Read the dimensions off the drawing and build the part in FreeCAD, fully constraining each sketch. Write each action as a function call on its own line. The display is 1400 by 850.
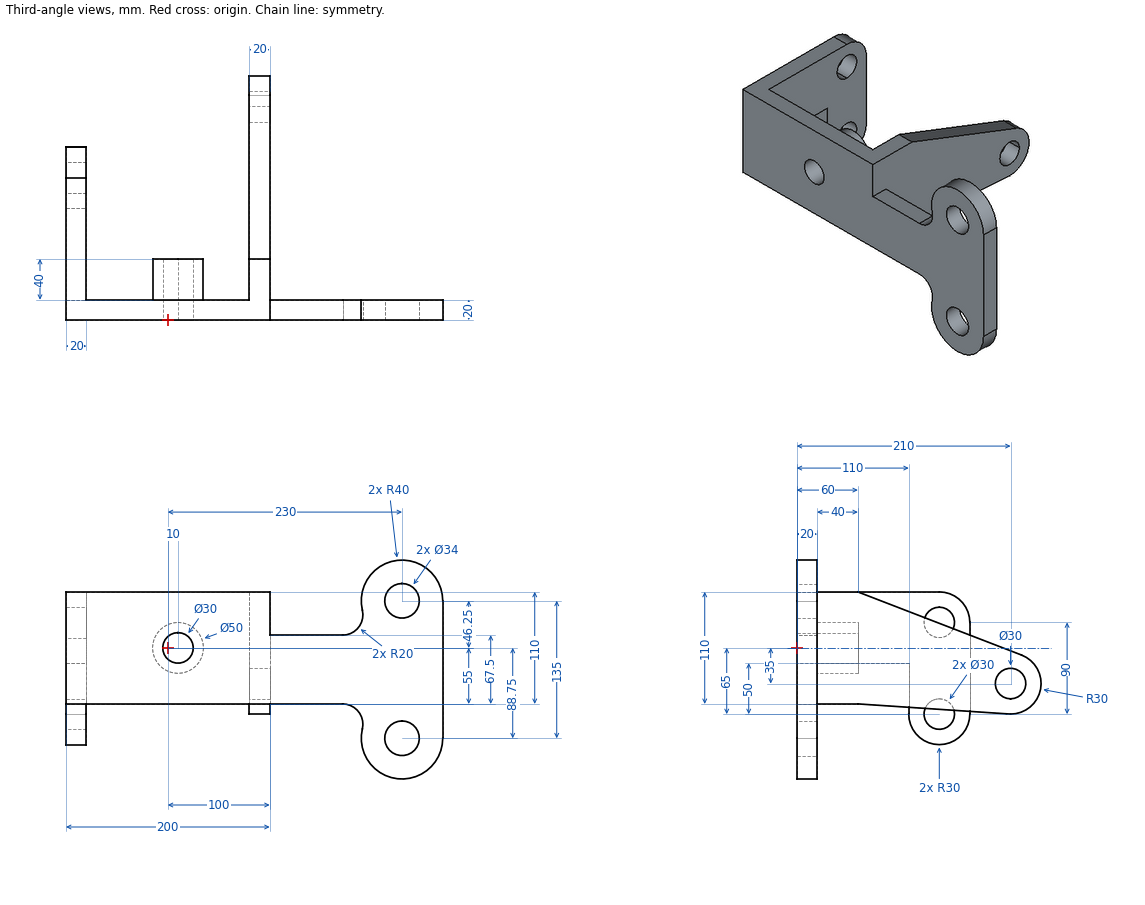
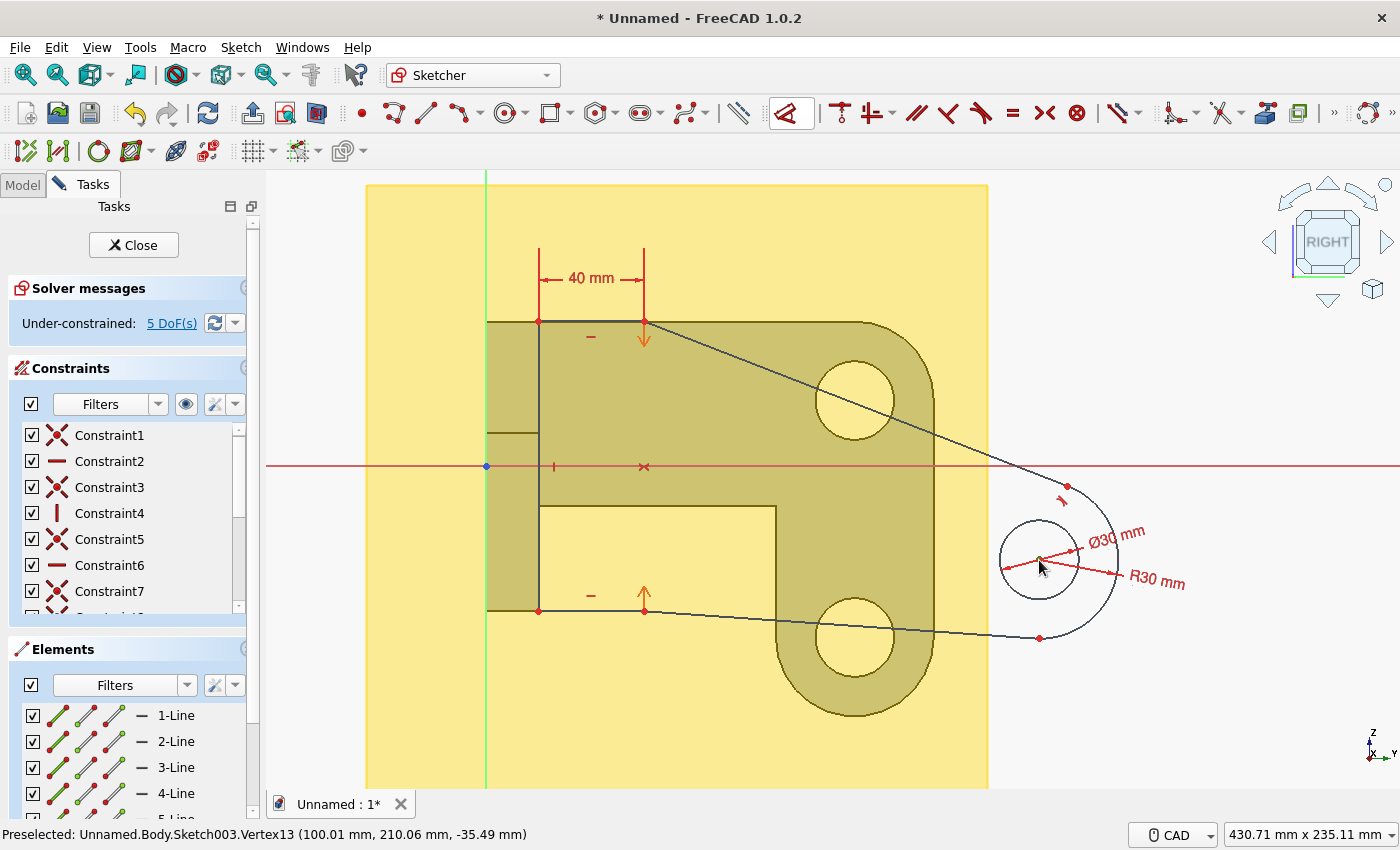
key(i)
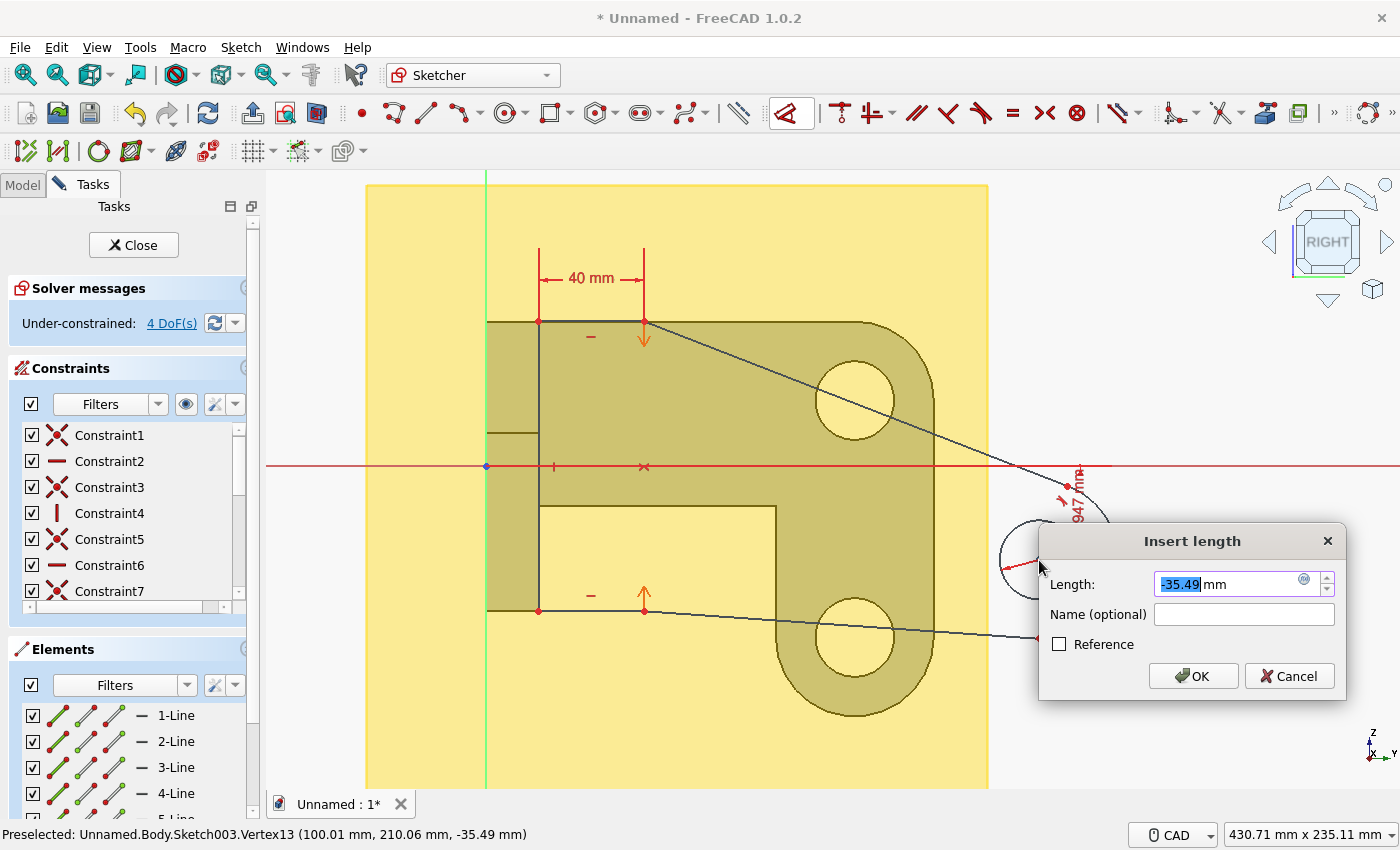
text(-35)
key(Return)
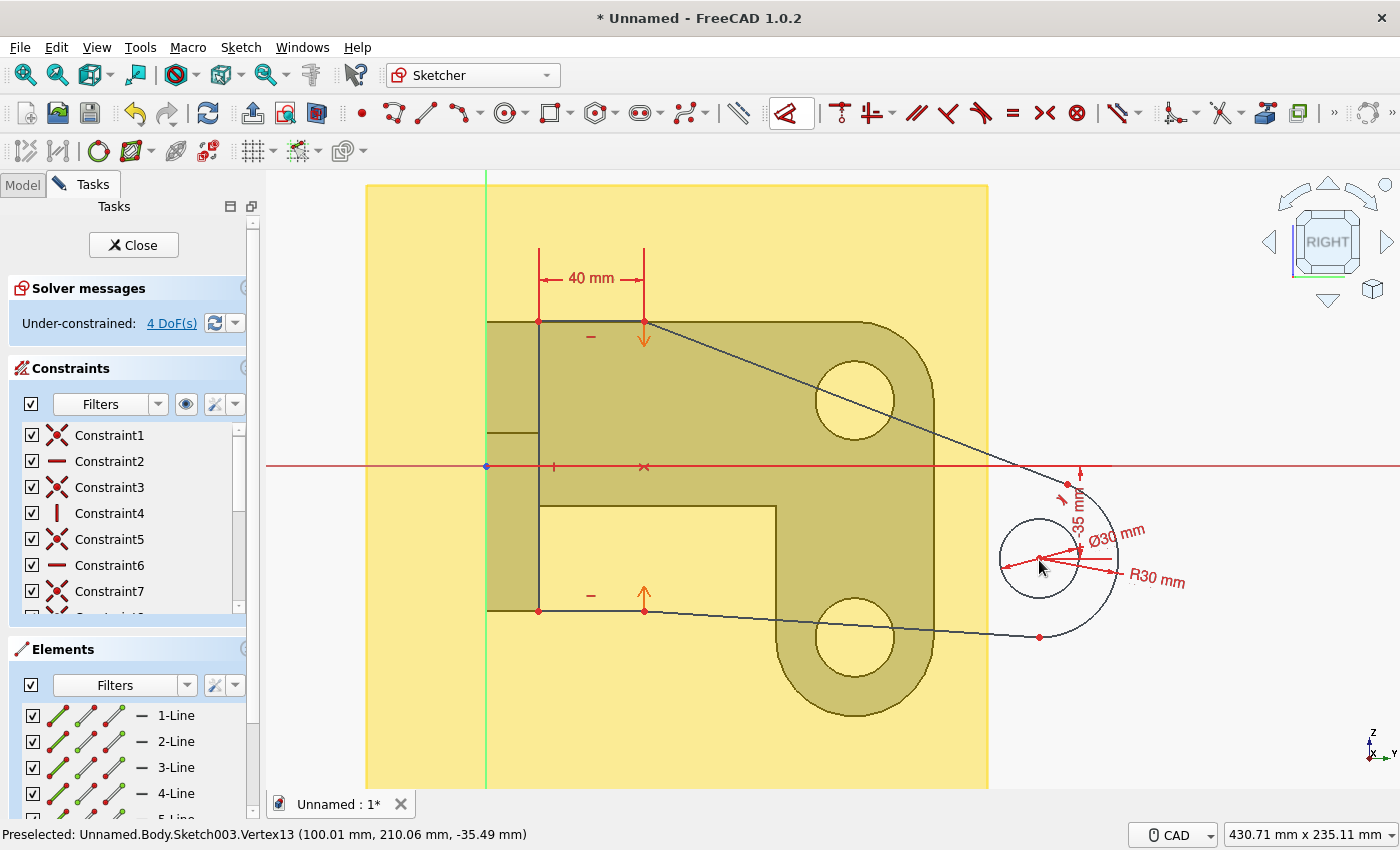
click(539, 408)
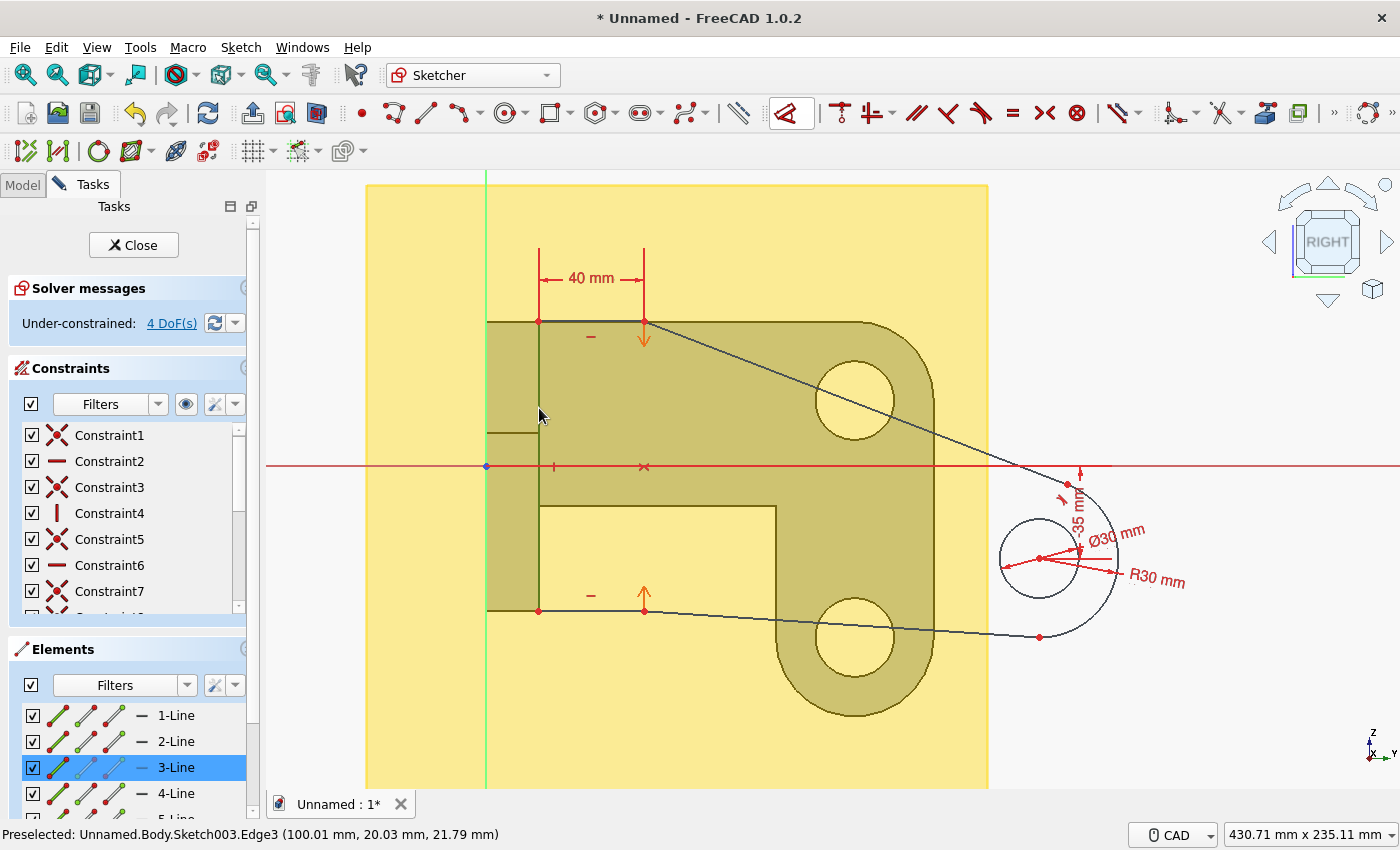
key(i)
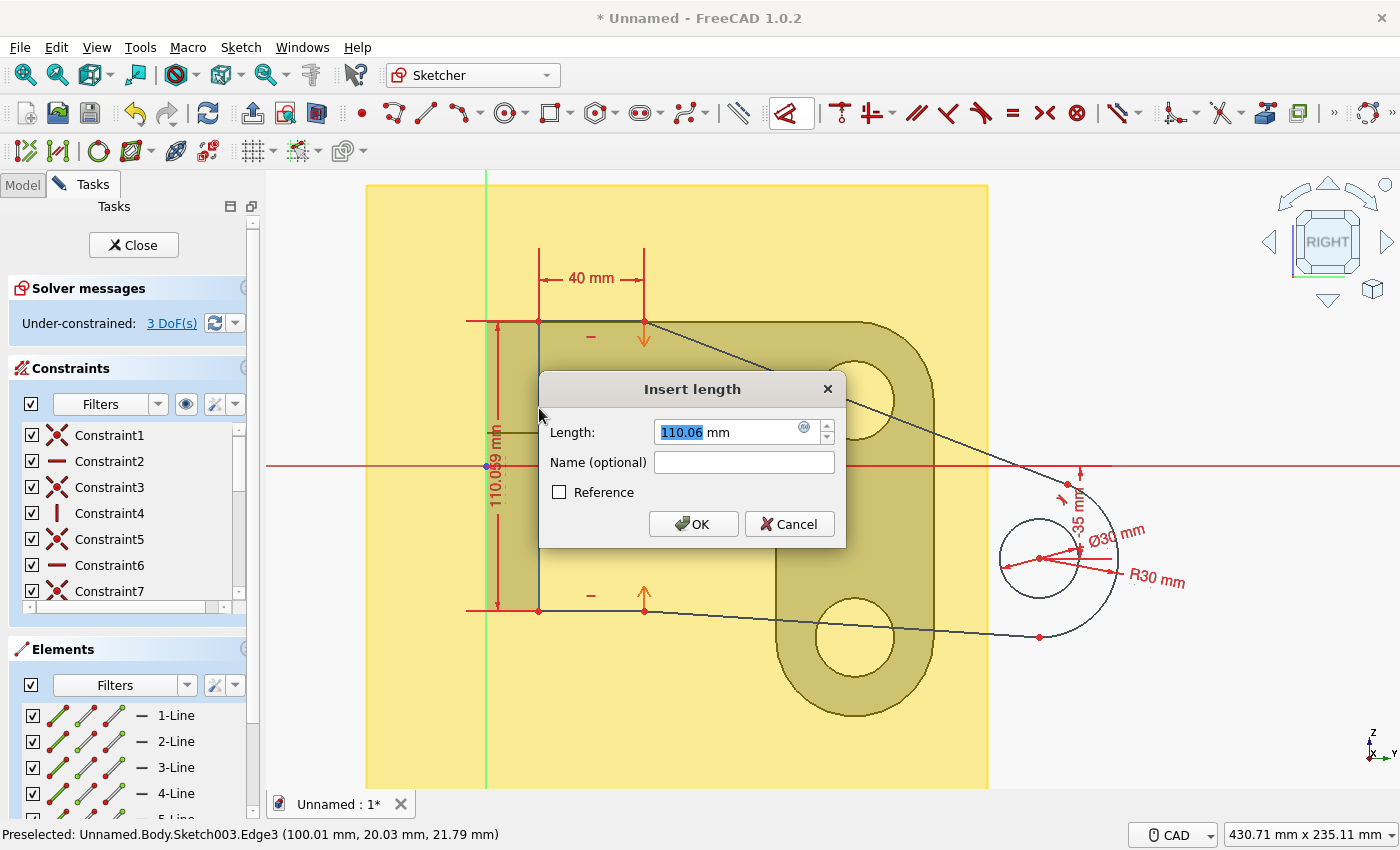
text(110)
key(Return)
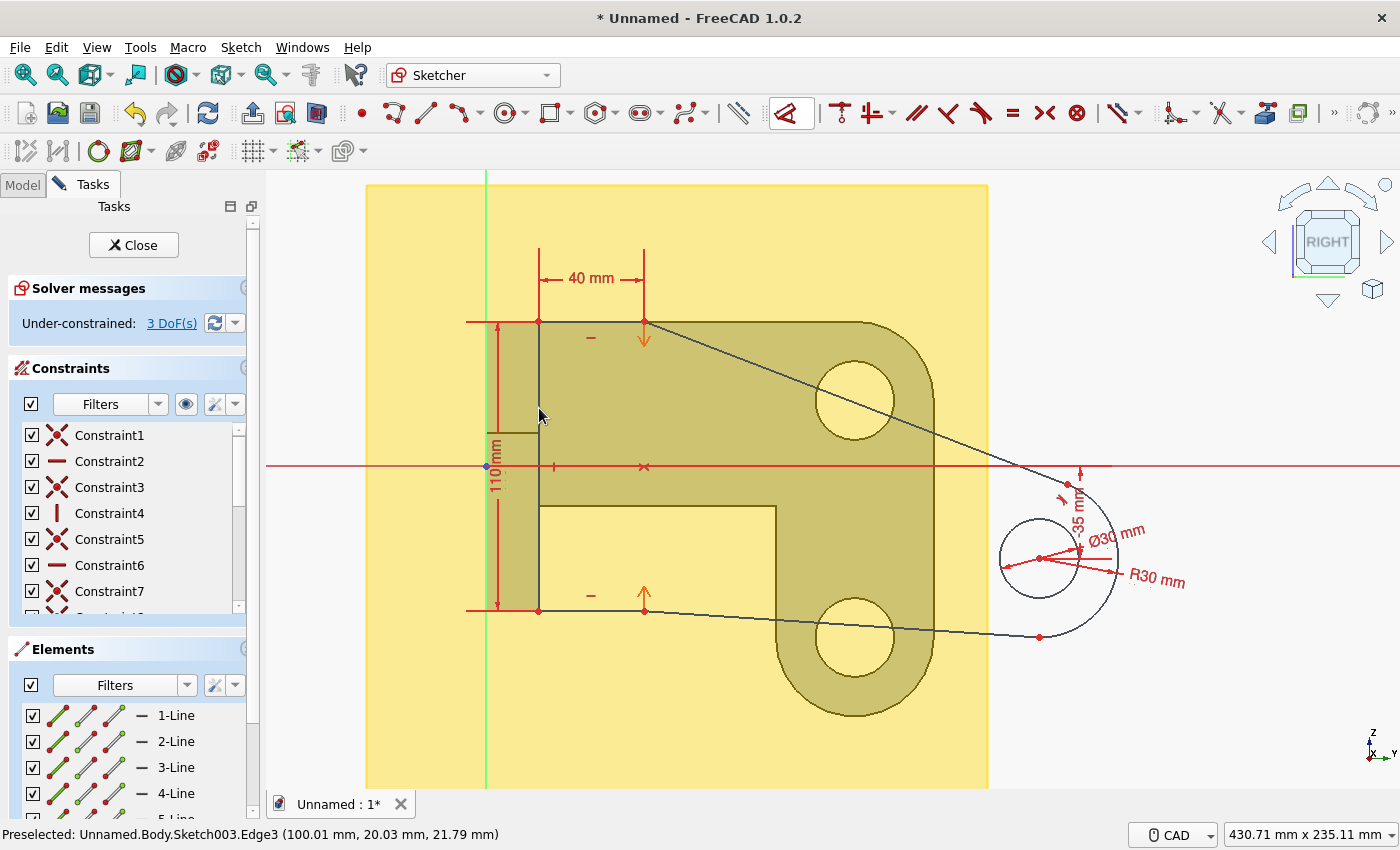
click(644, 322)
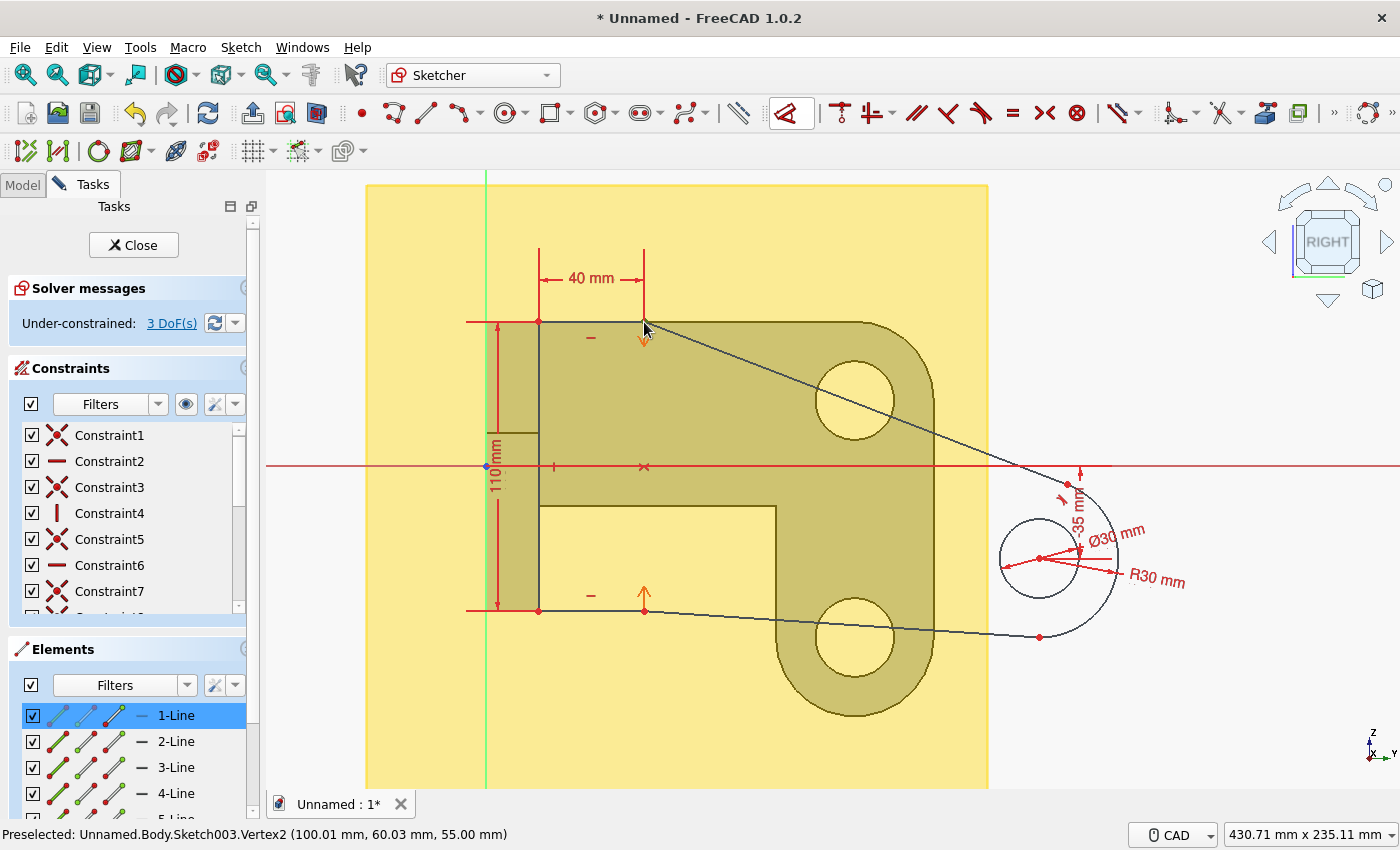
key(l)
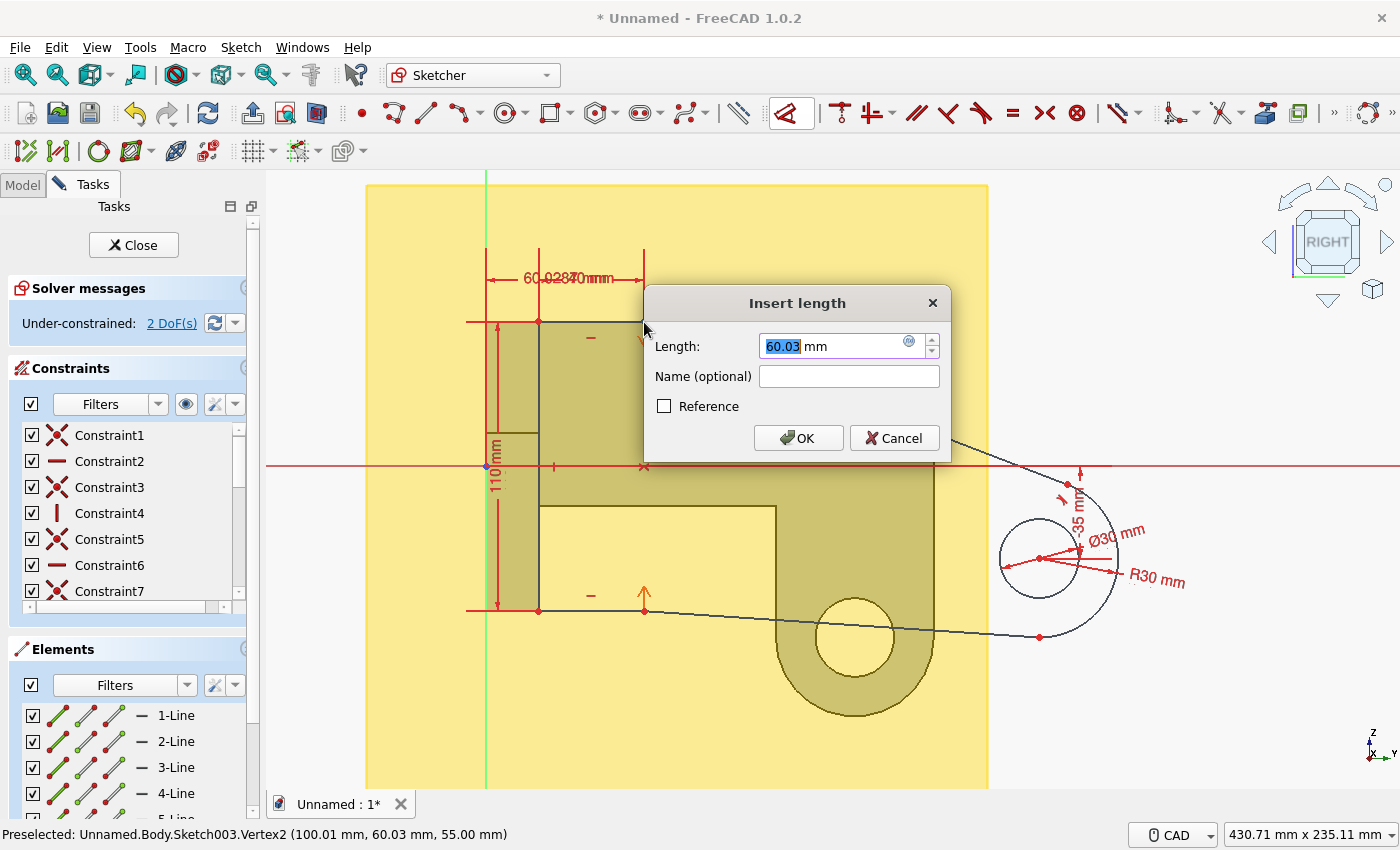
text(60)
key(Return)